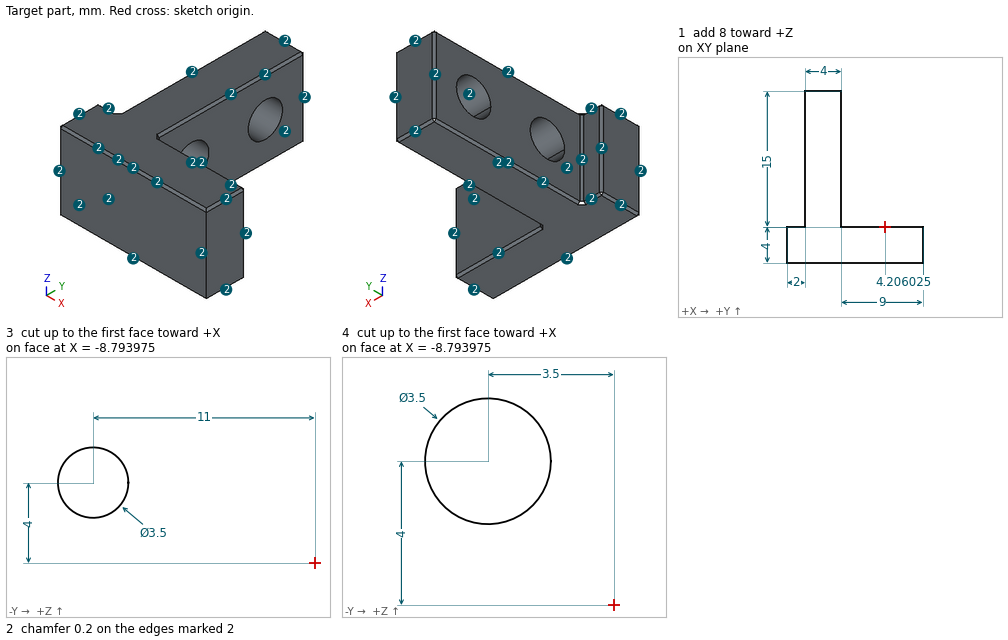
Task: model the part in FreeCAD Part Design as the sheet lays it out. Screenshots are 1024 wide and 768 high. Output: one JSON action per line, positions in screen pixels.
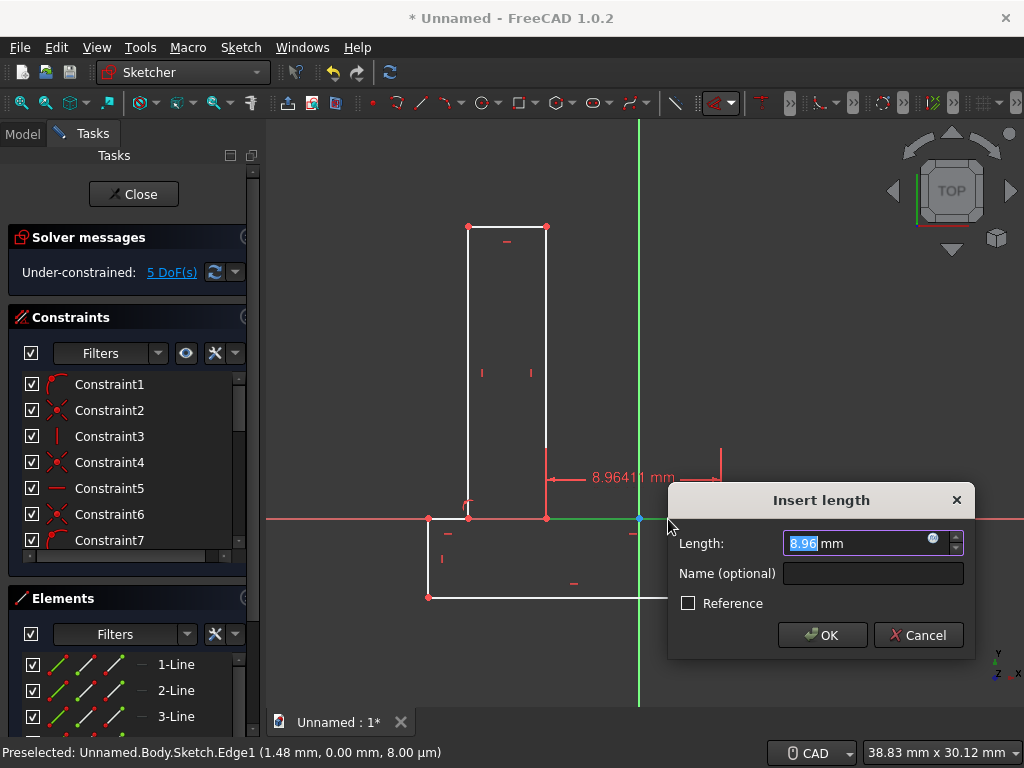
{"action": "type", "text": "9"}
{"action": "key", "text": "Return"}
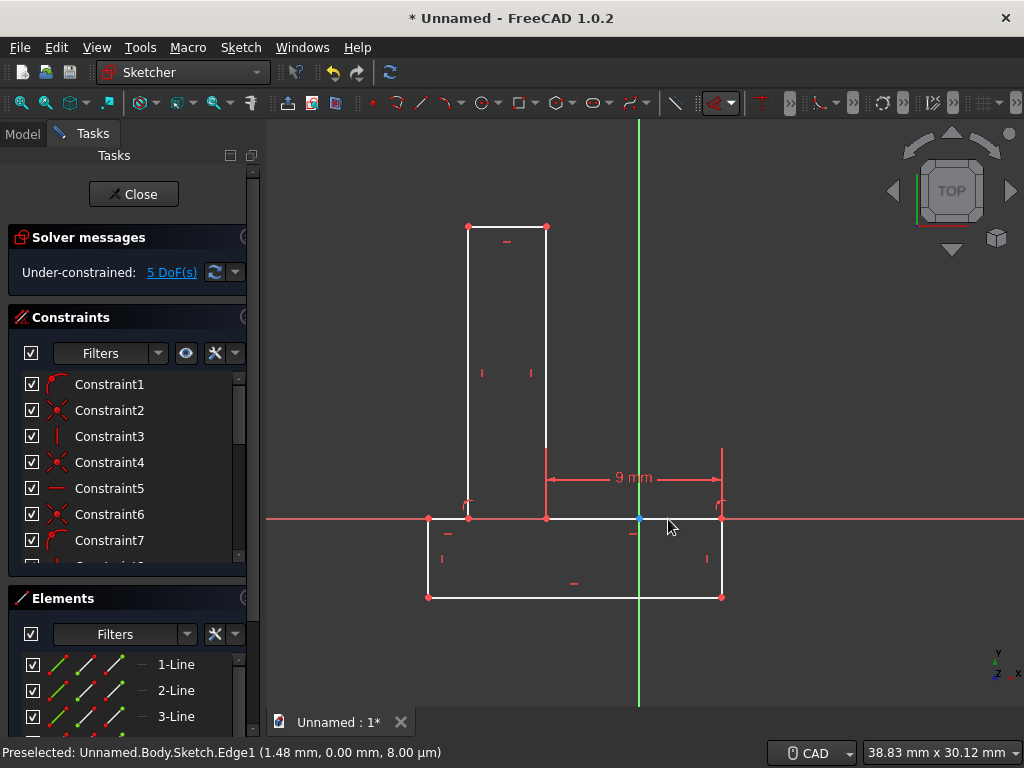
{"action": "left_click", "coordinate": [523, 227]}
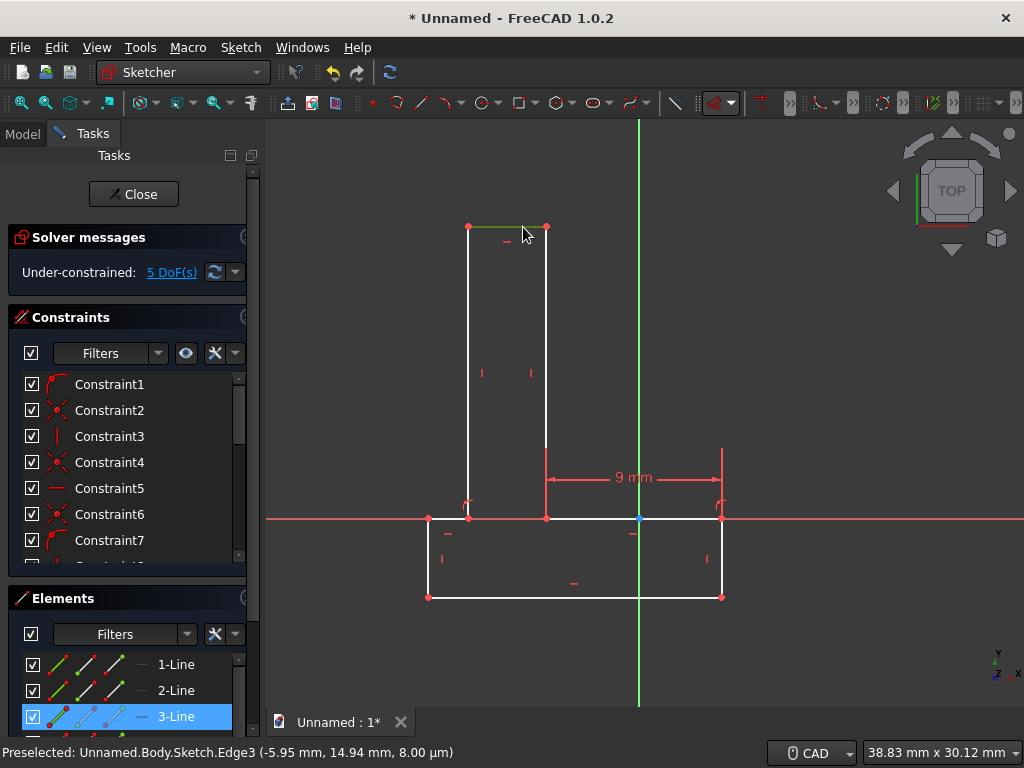
{"action": "left_click", "coordinate": [734, 104]}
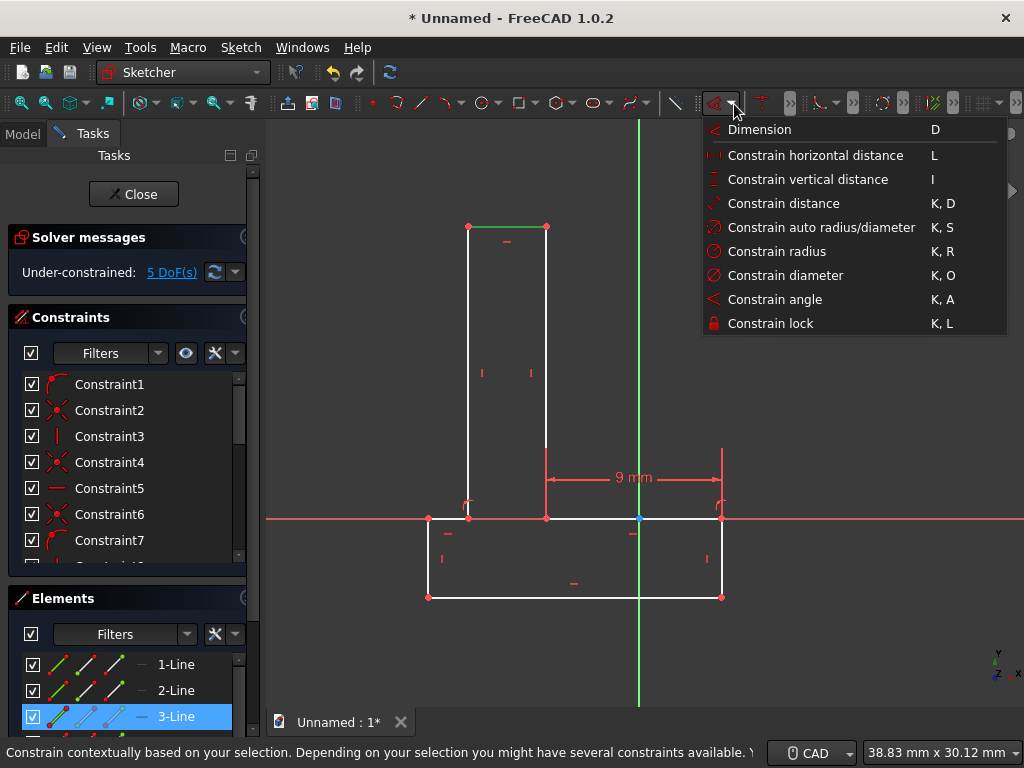
{"action": "left_click", "coordinate": [855, 155]}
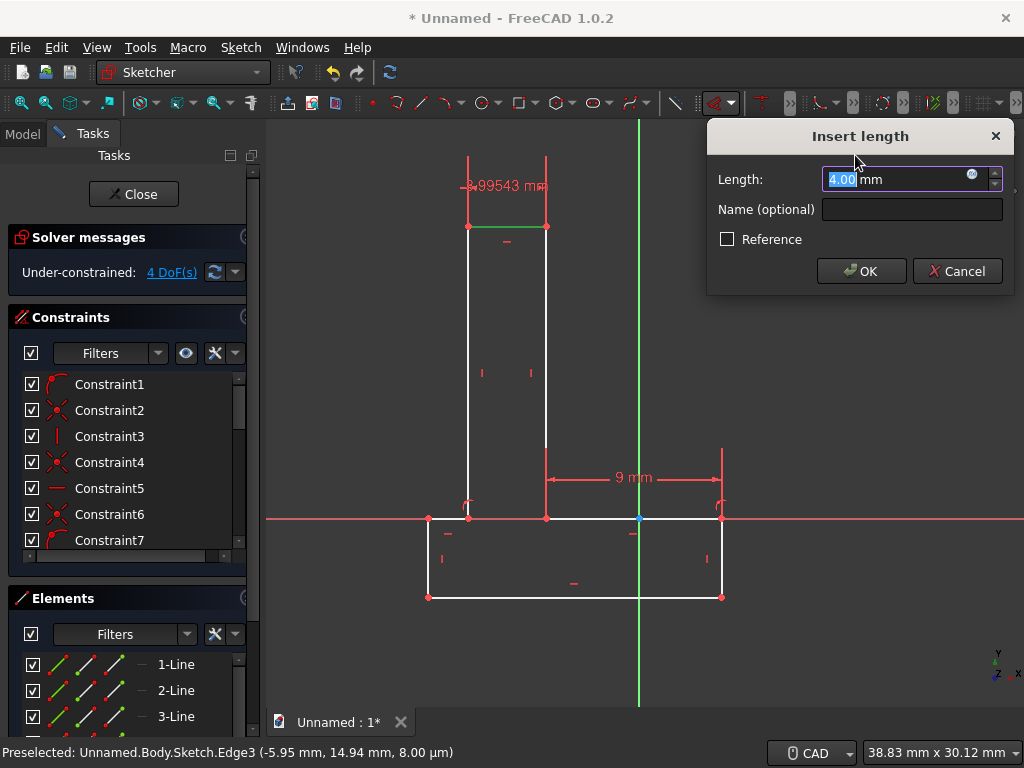
{"action": "type", "text": "4"}
{"action": "key", "text": "Return"}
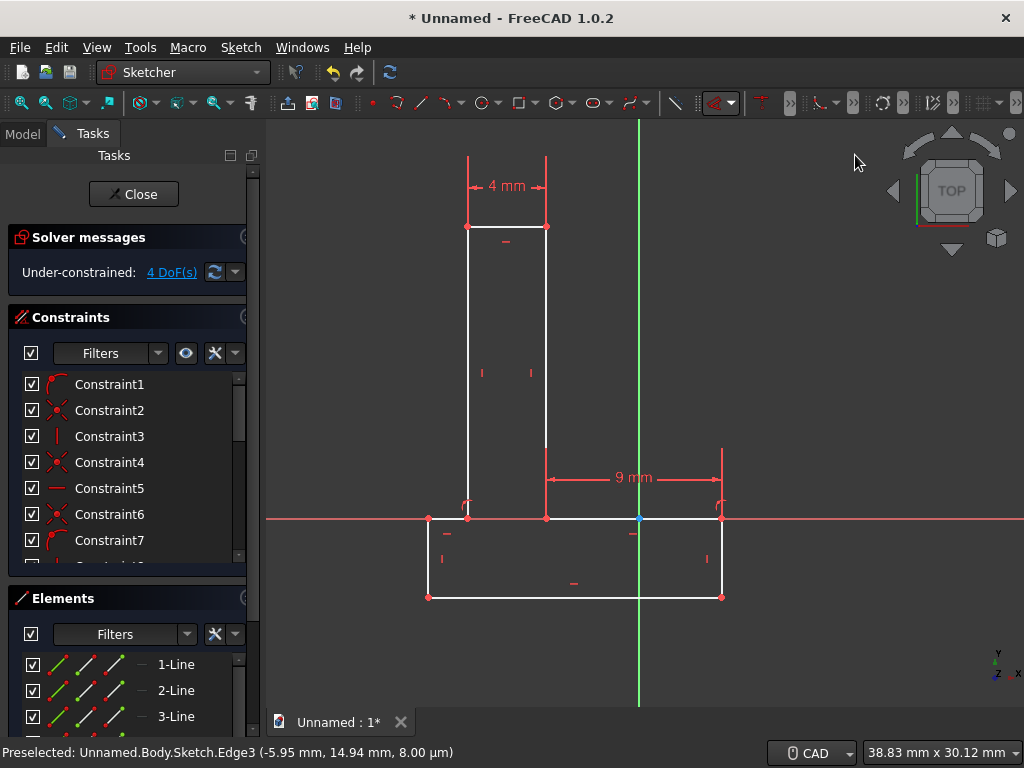
{"action": "left_click", "coordinate": [456, 519]}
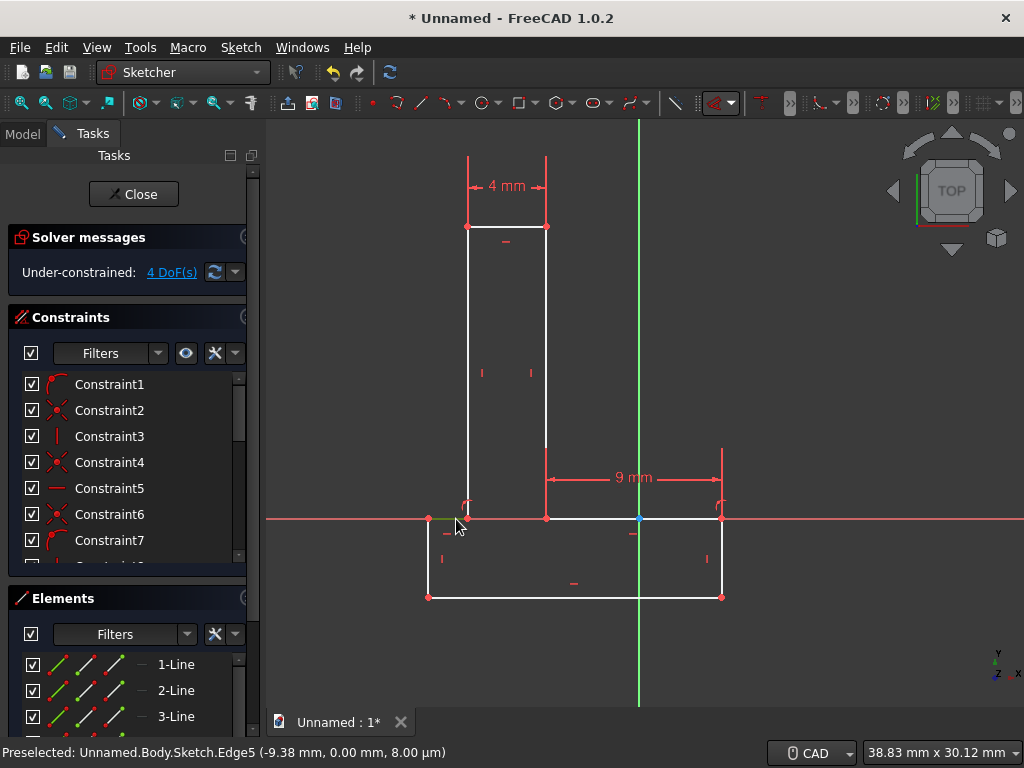
{"action": "left_click", "coordinate": [734, 104]}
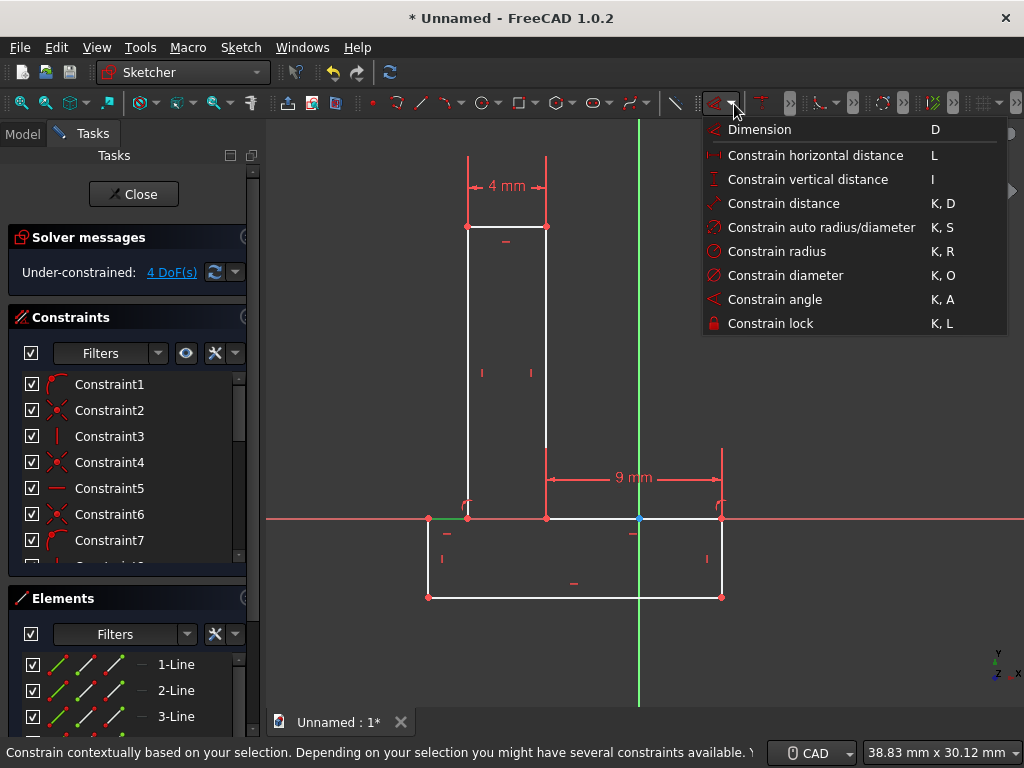
{"action": "left_click", "coordinate": [855, 155]}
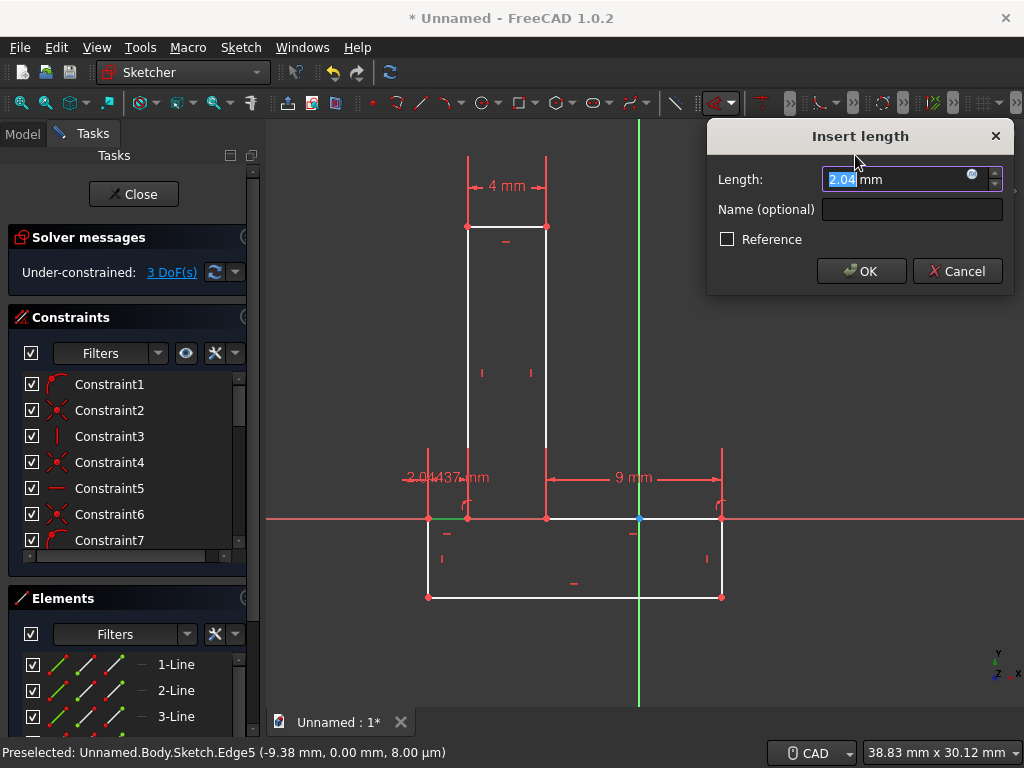
{"action": "type", "text": "2"}
{"action": "key", "text": "Return"}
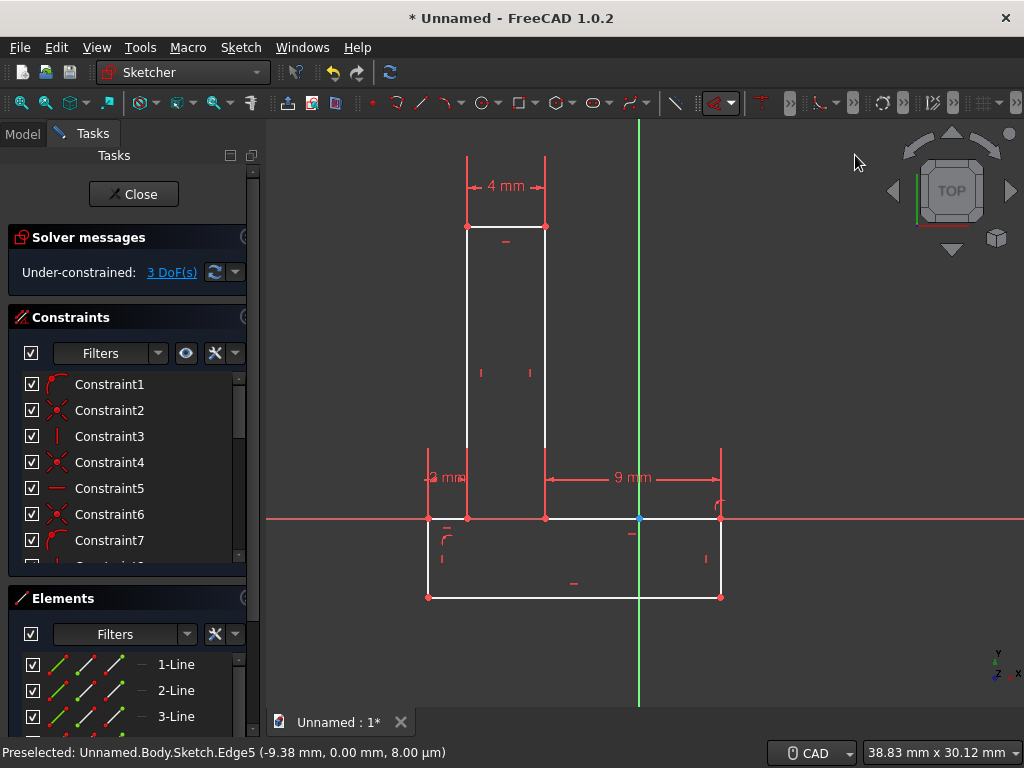
{"action": "left_click", "coordinate": [428, 543]}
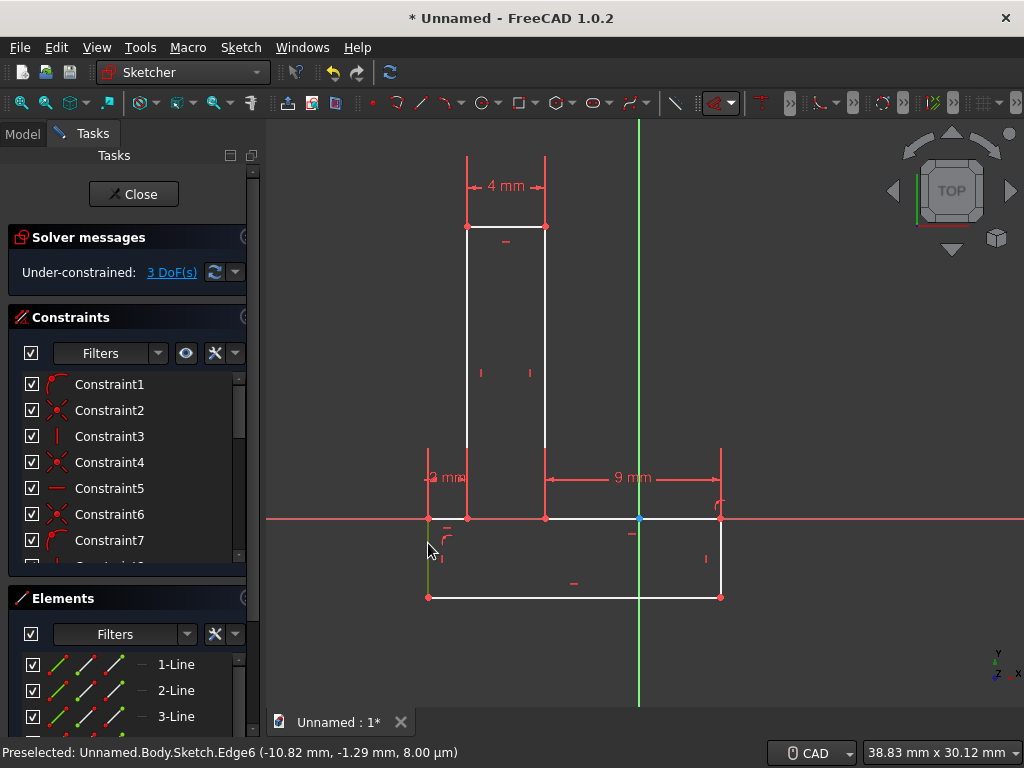
{"action": "left_click", "coordinate": [734, 104]}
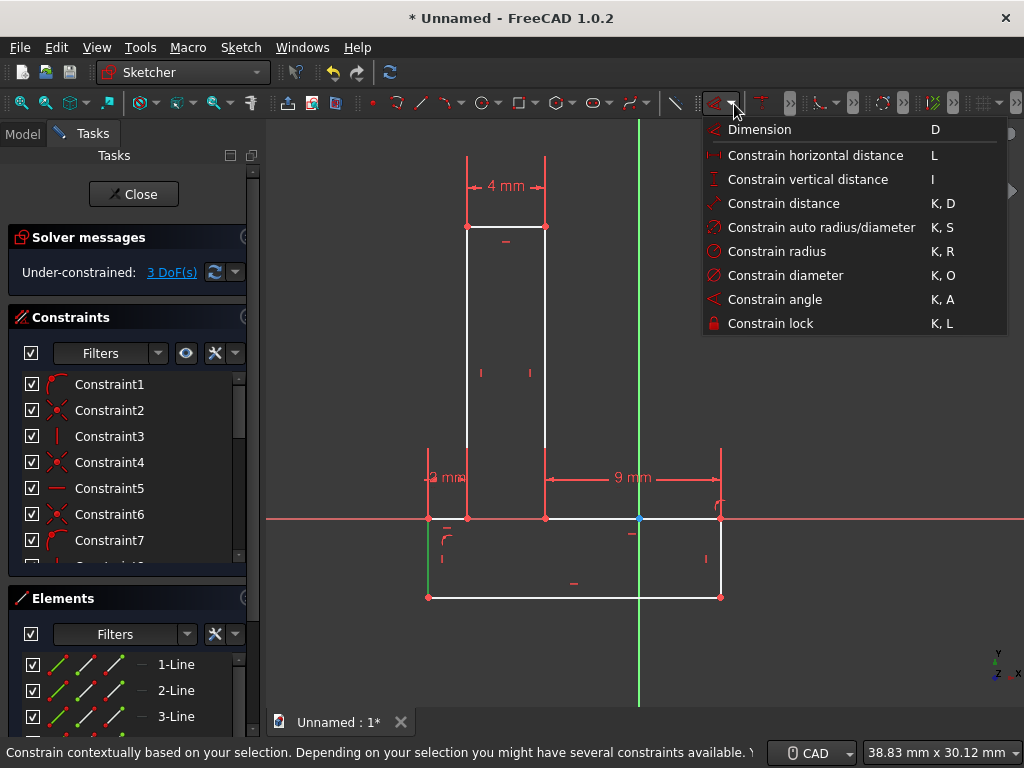
{"action": "left_click", "coordinate": [855, 179]}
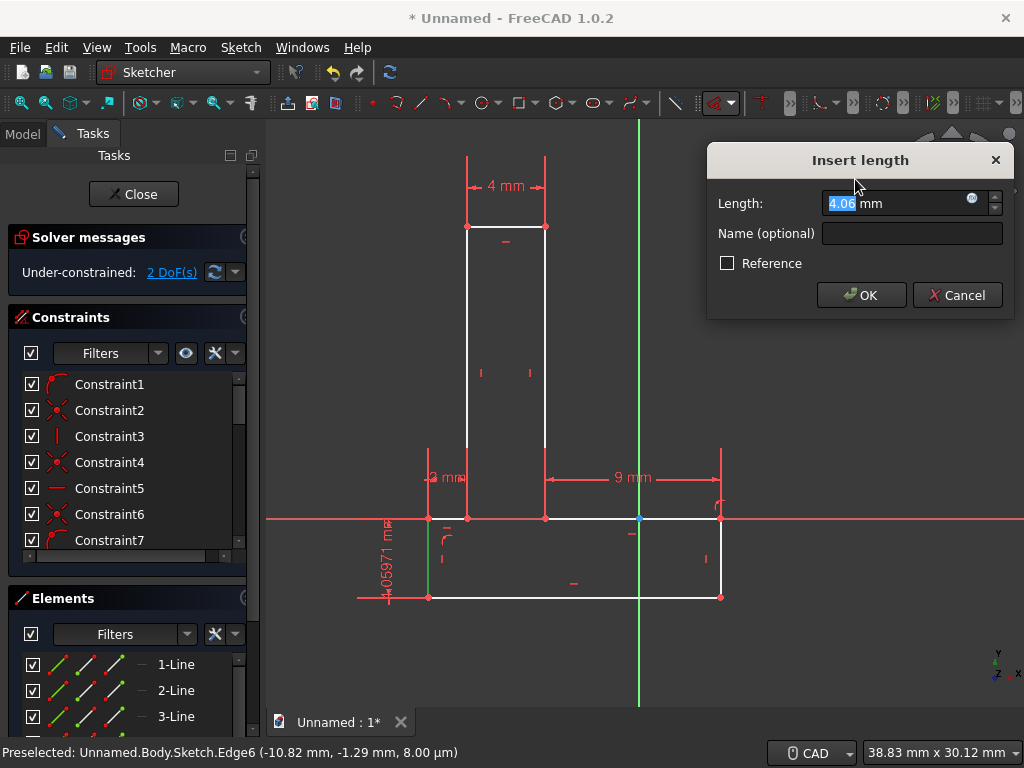
{"action": "type", "text": "4"}
{"action": "key", "text": "Return"}